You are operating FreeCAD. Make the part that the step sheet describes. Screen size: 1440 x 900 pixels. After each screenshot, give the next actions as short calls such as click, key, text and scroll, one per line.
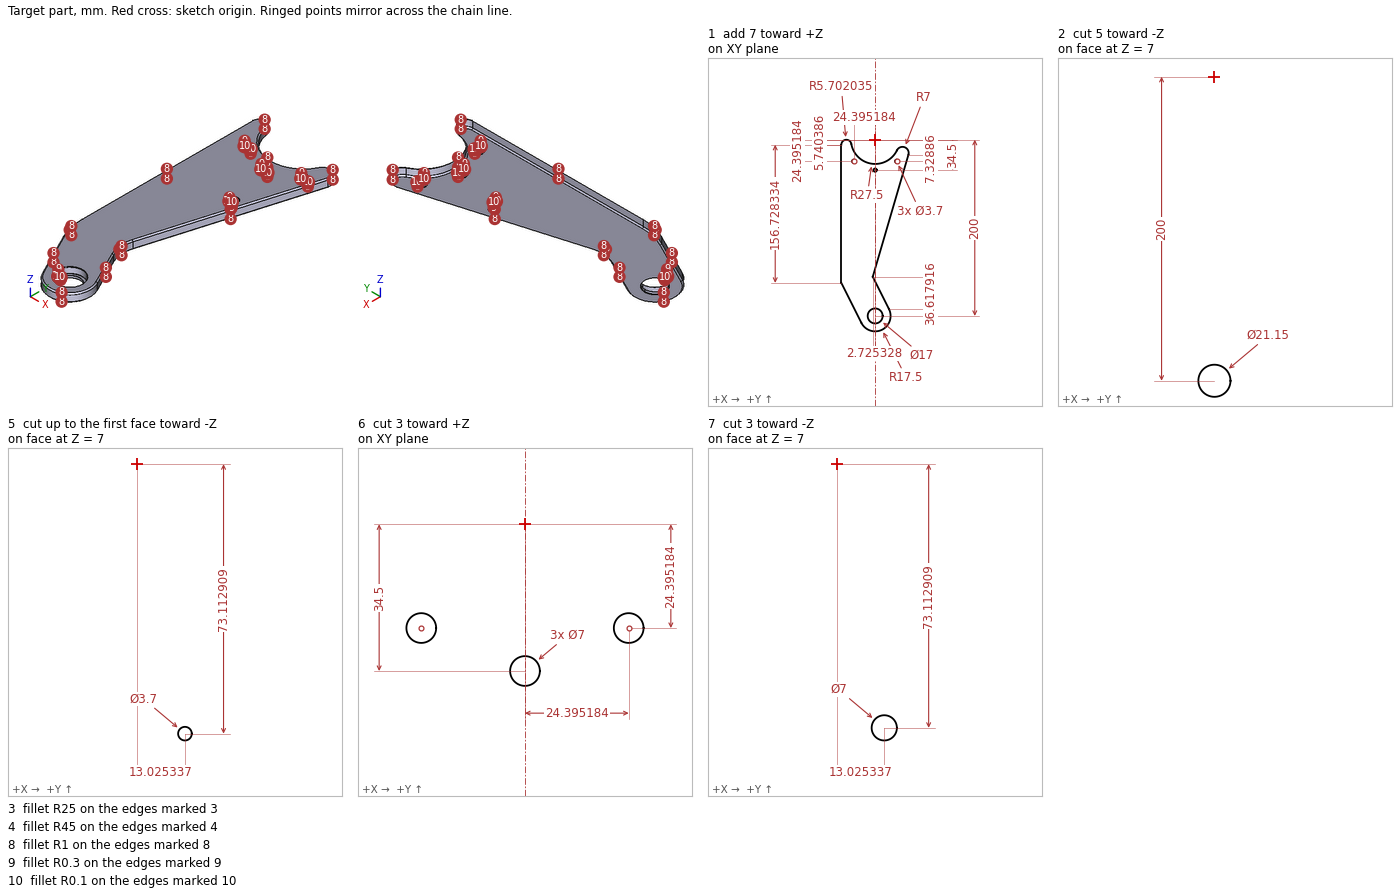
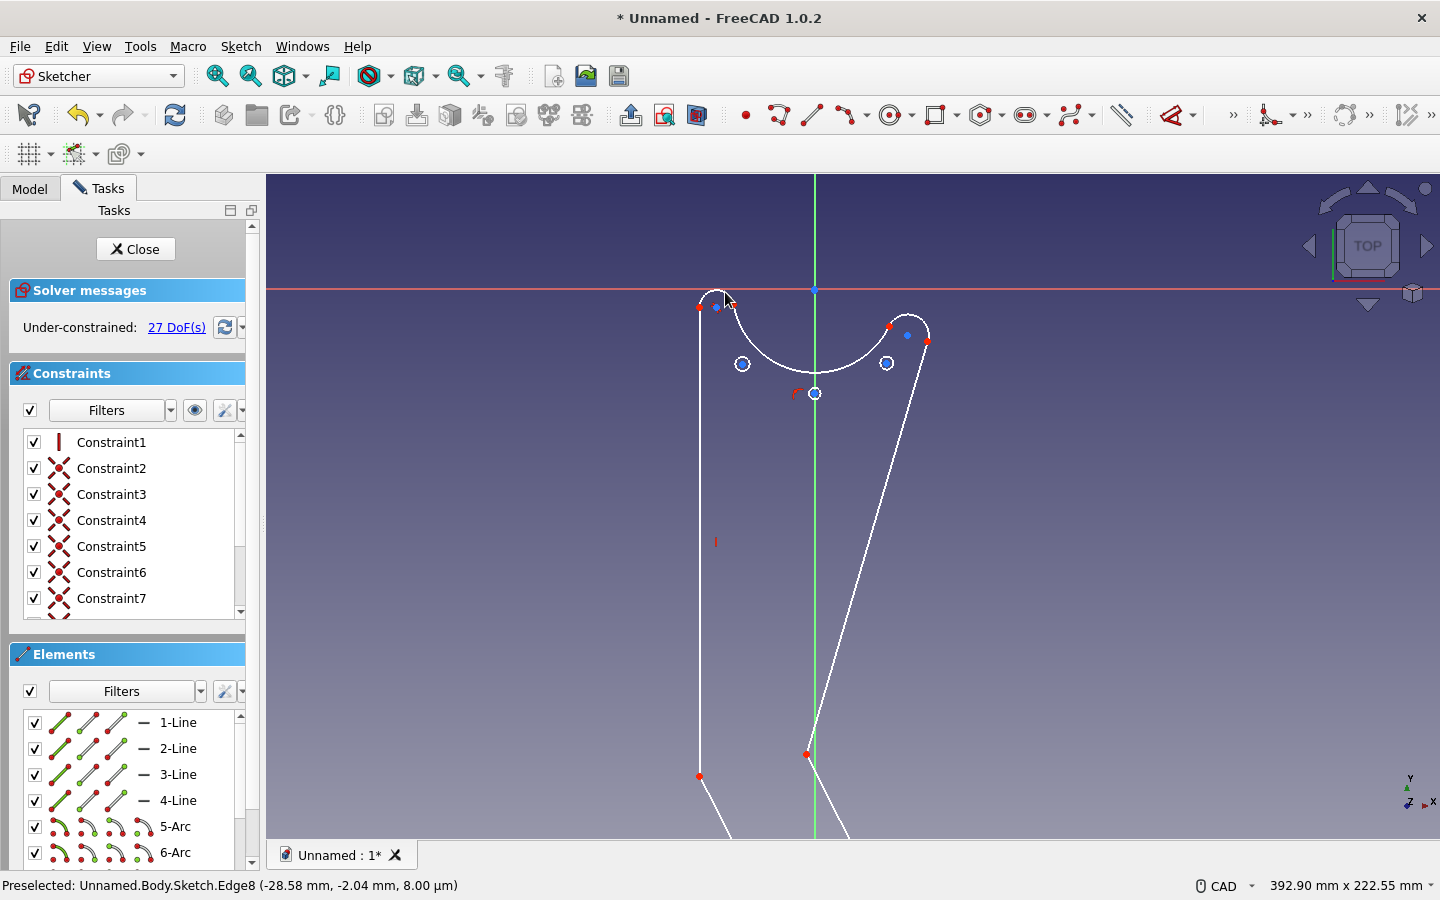
click(713, 803)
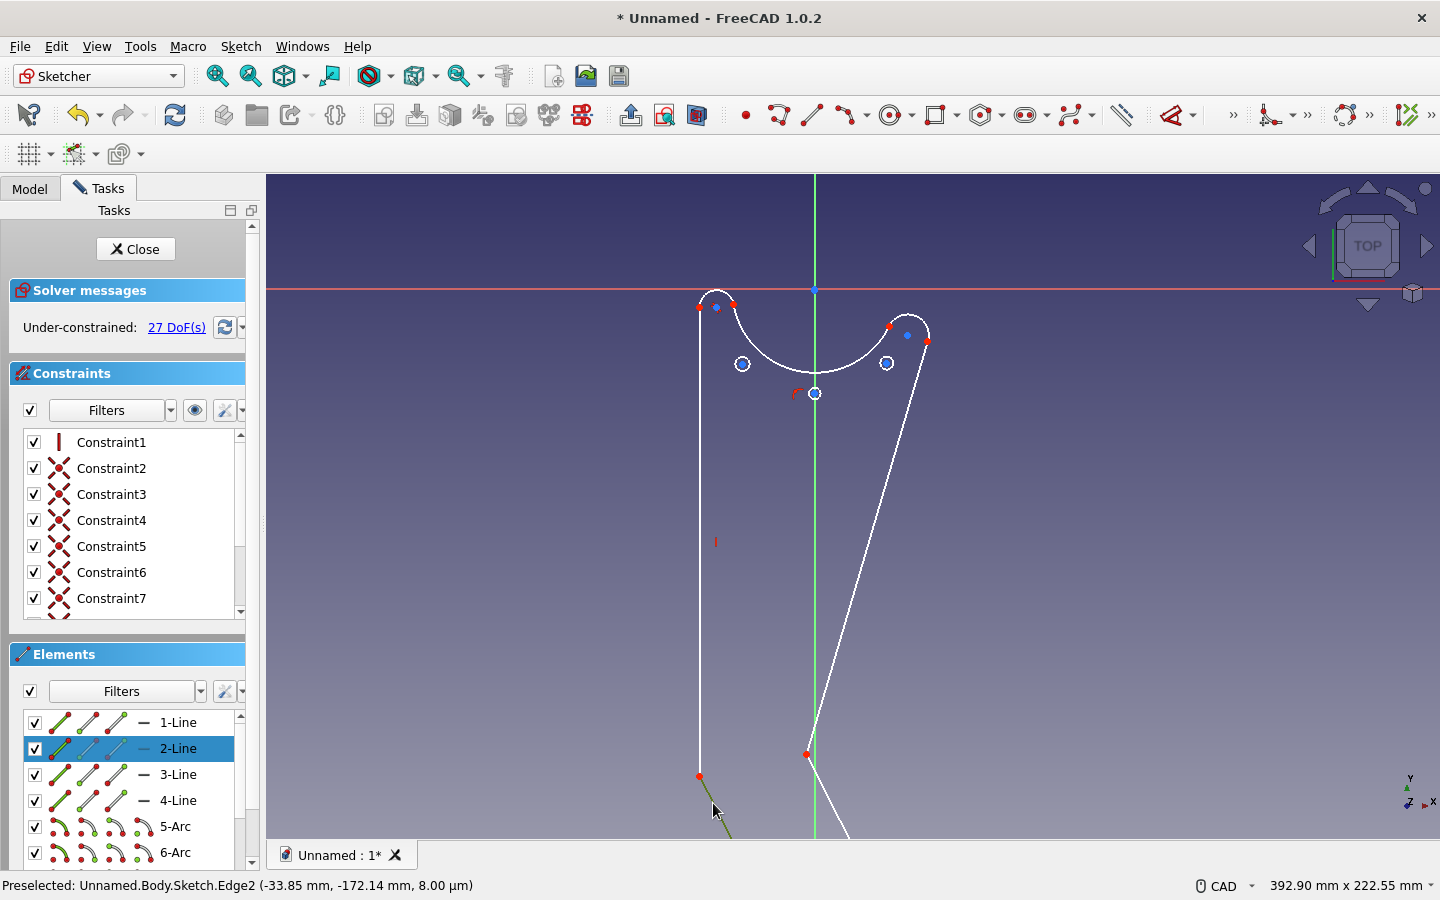
scroll(725, 293, down, 2)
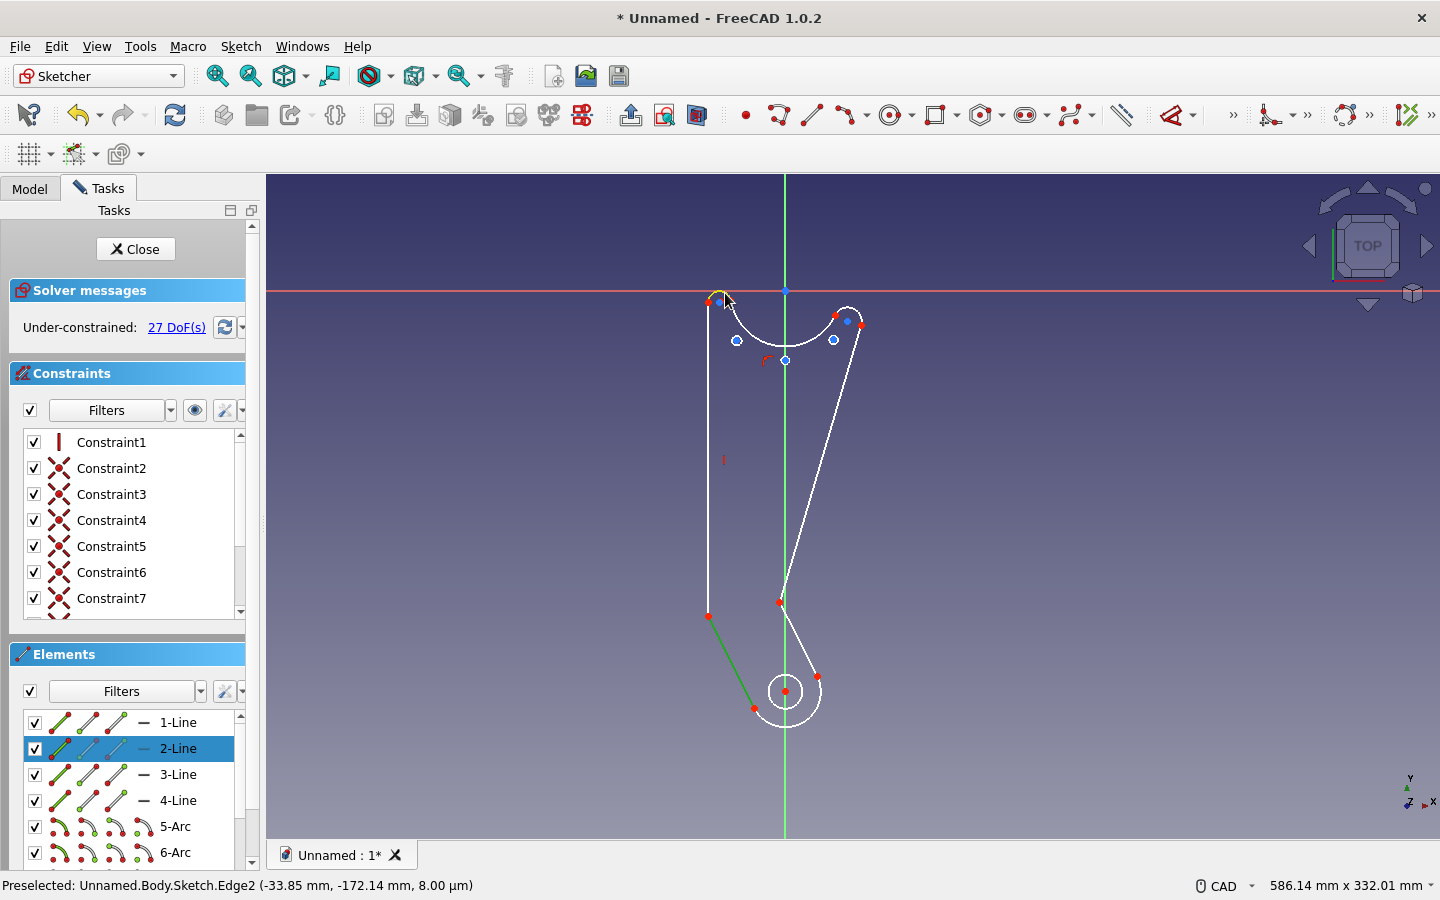
click(817, 708)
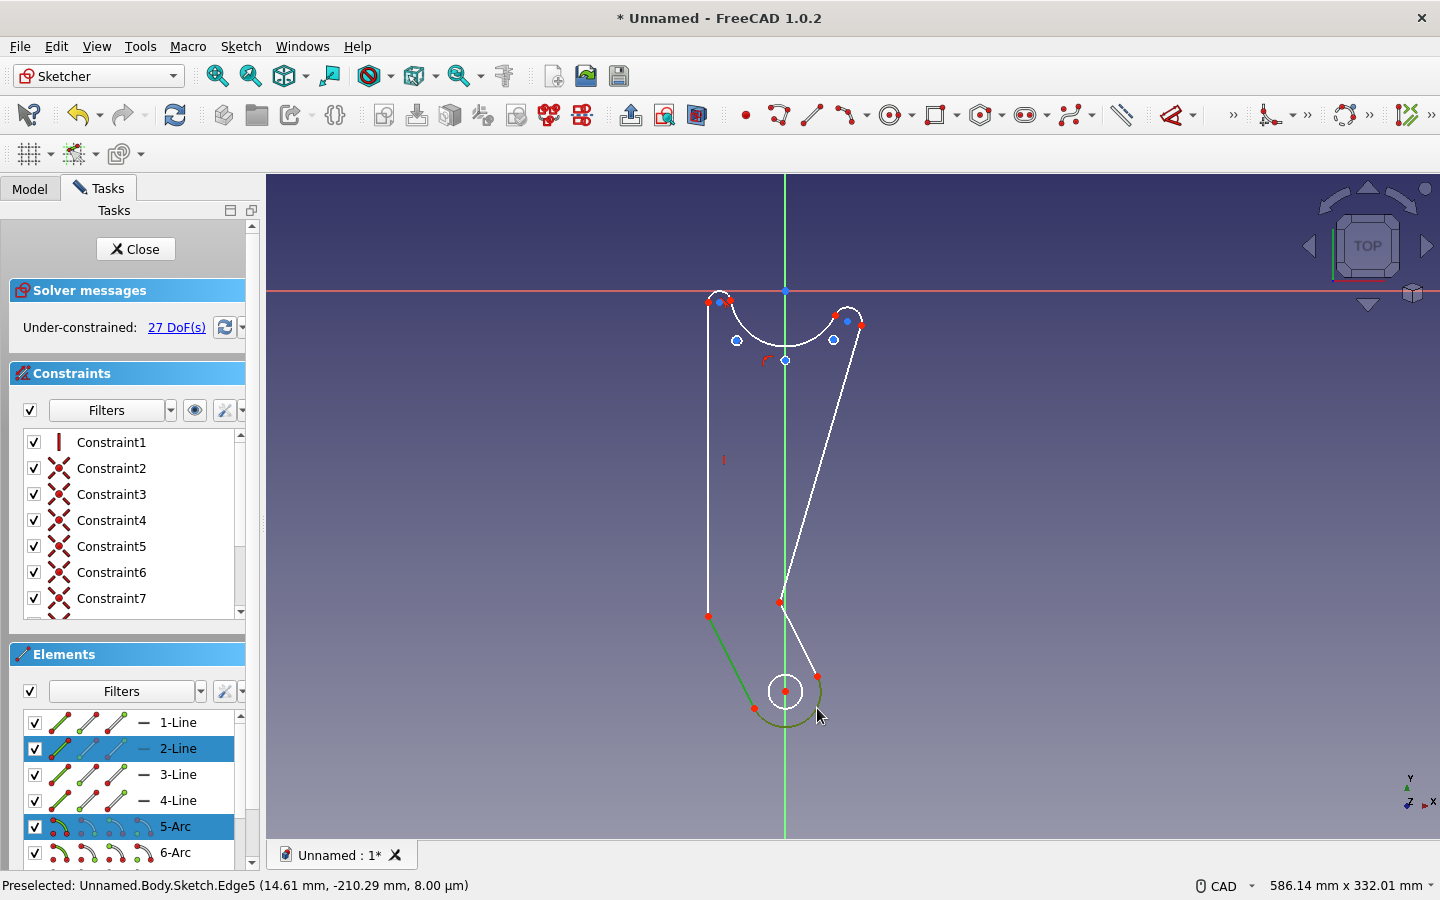
key(t)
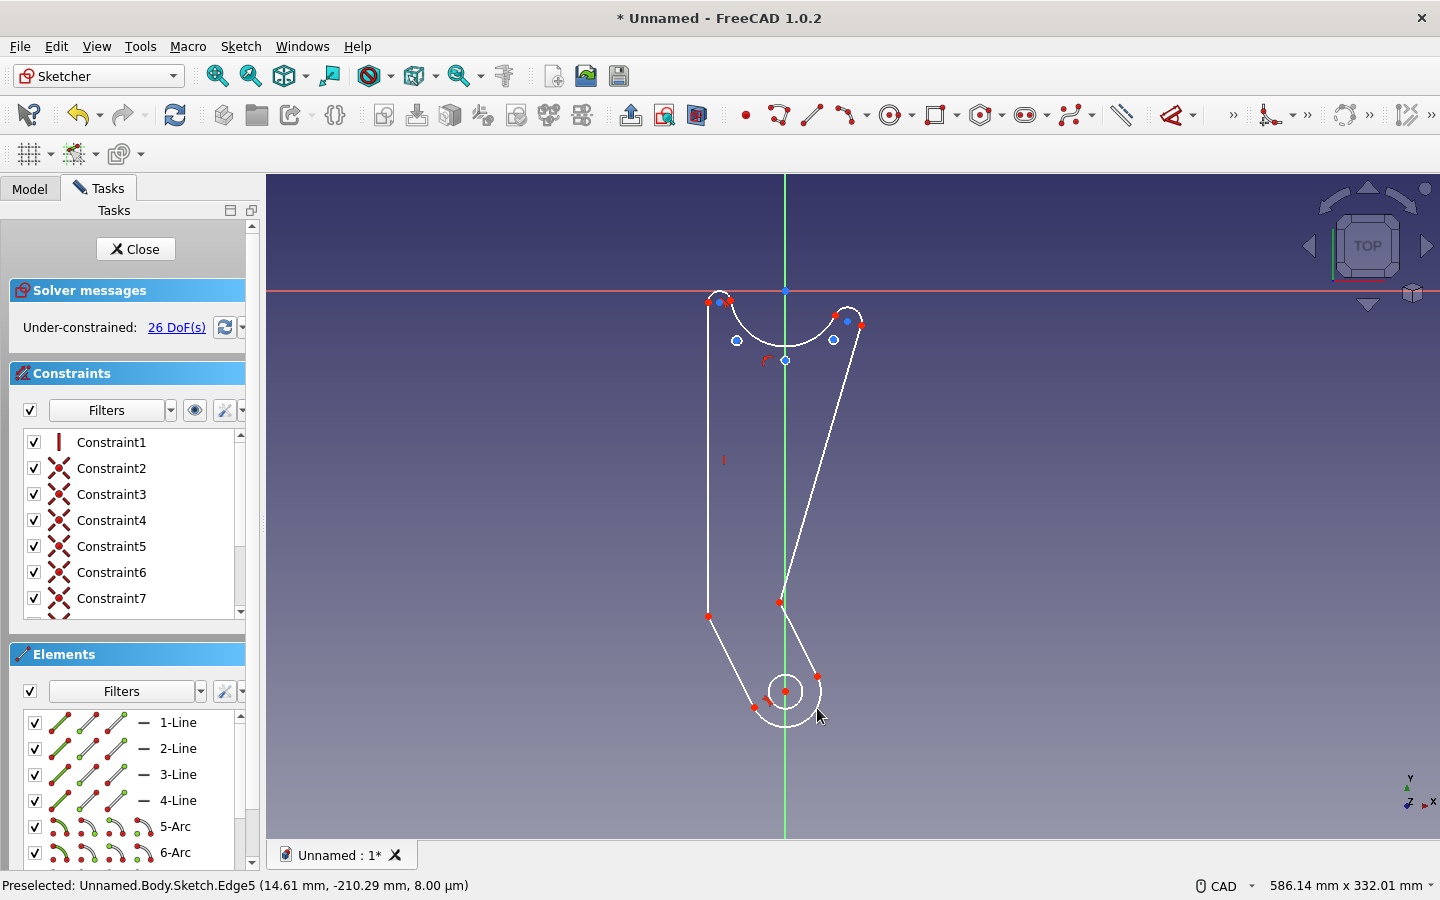
click(806, 654)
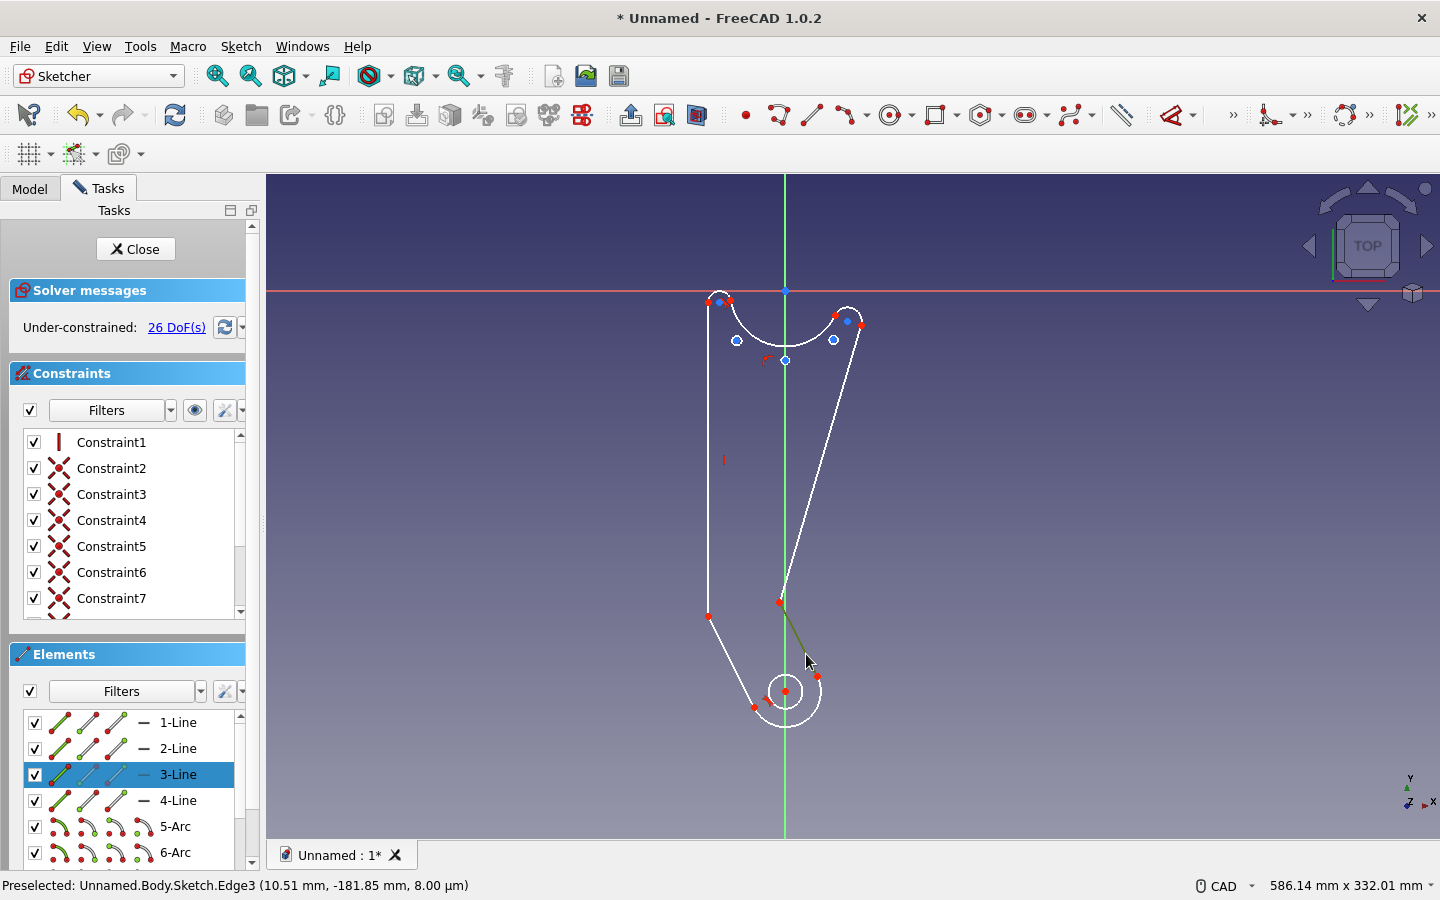
click(817, 708)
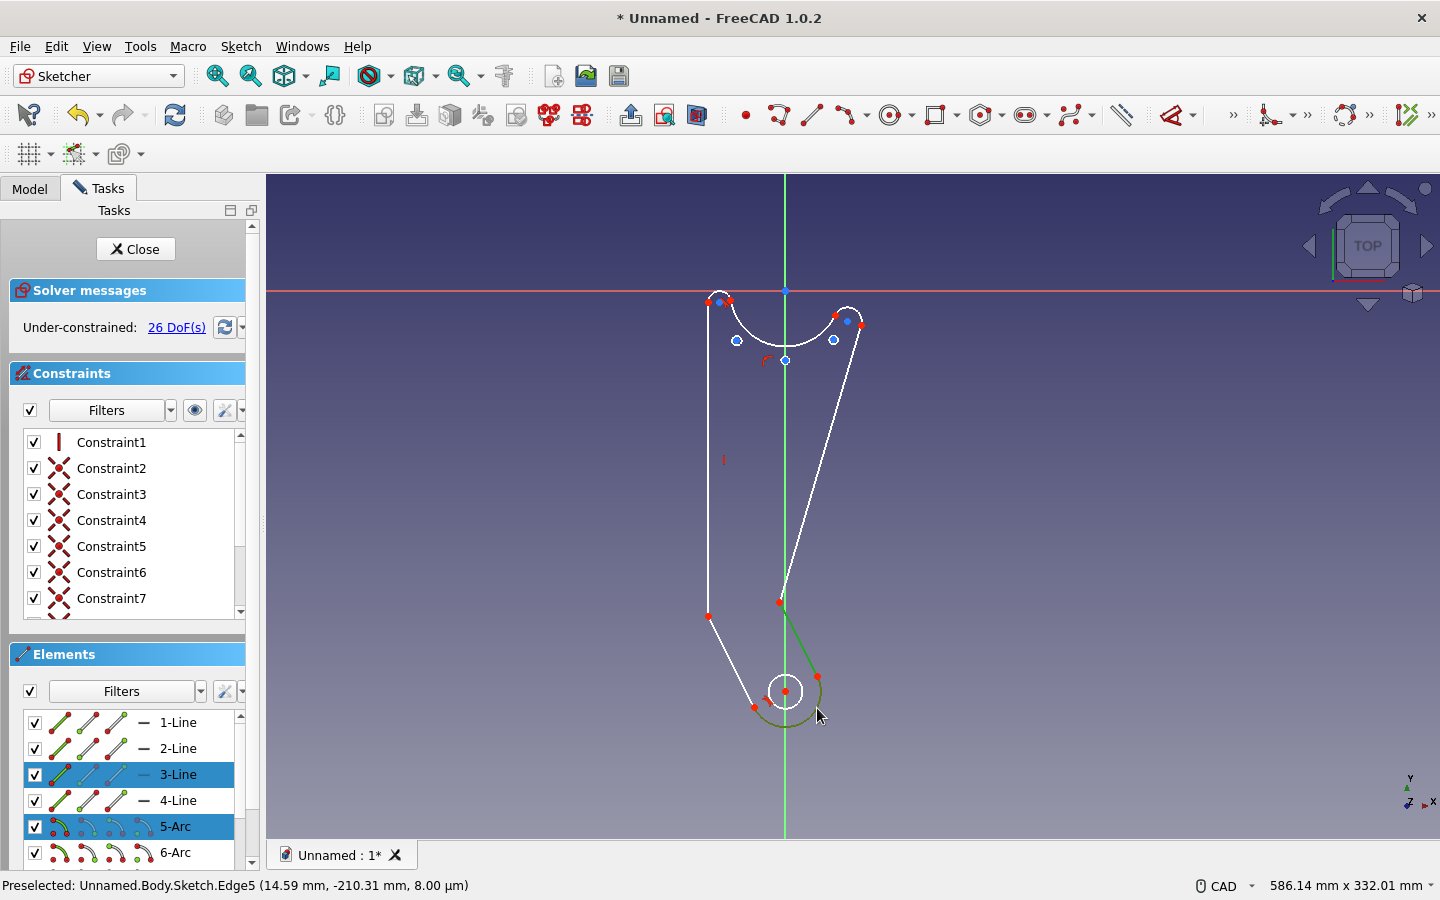
key(t)